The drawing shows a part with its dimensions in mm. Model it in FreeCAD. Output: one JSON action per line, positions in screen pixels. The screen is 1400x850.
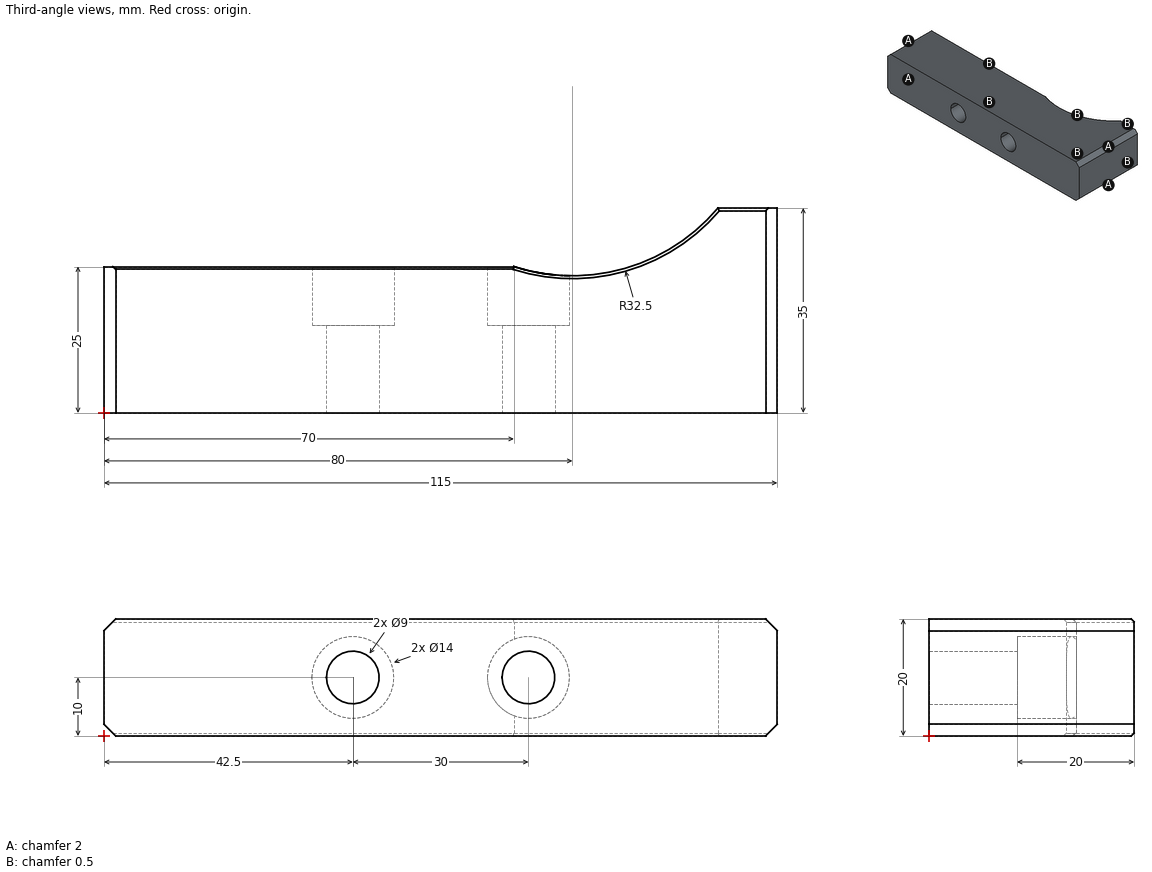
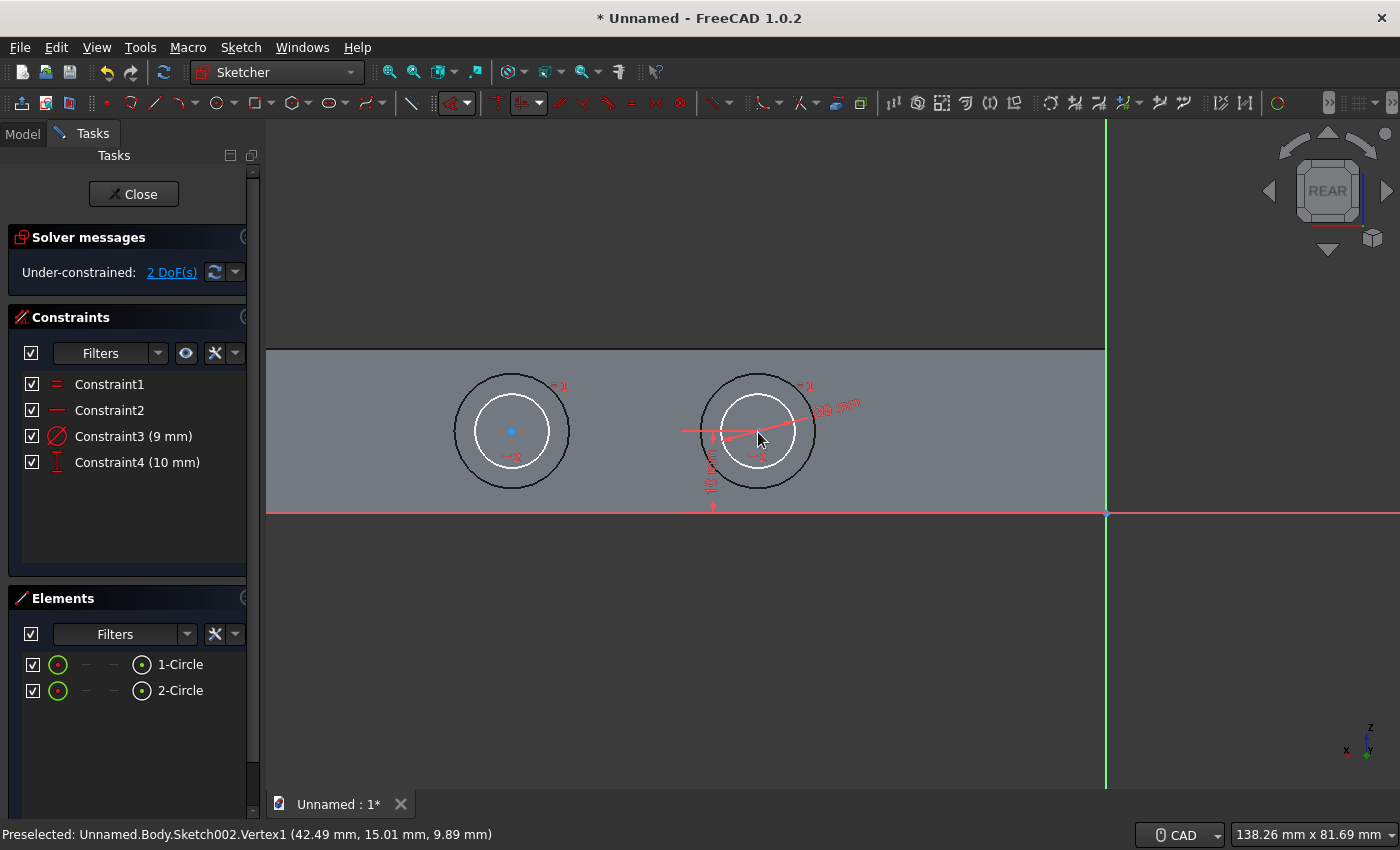
{"action": "left_click", "coordinate": [758, 431]}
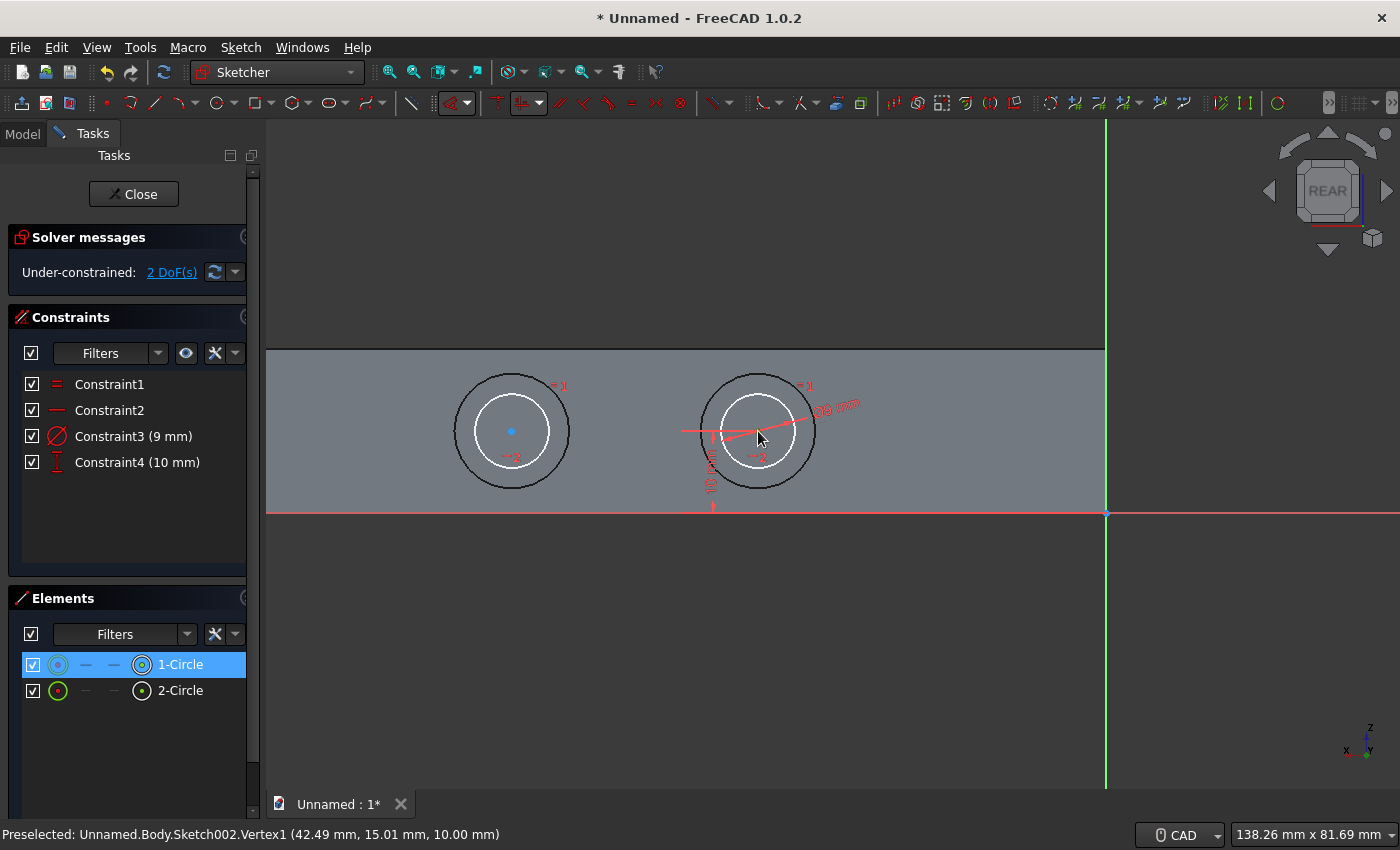
{"action": "left_click", "coordinate": [512, 431]}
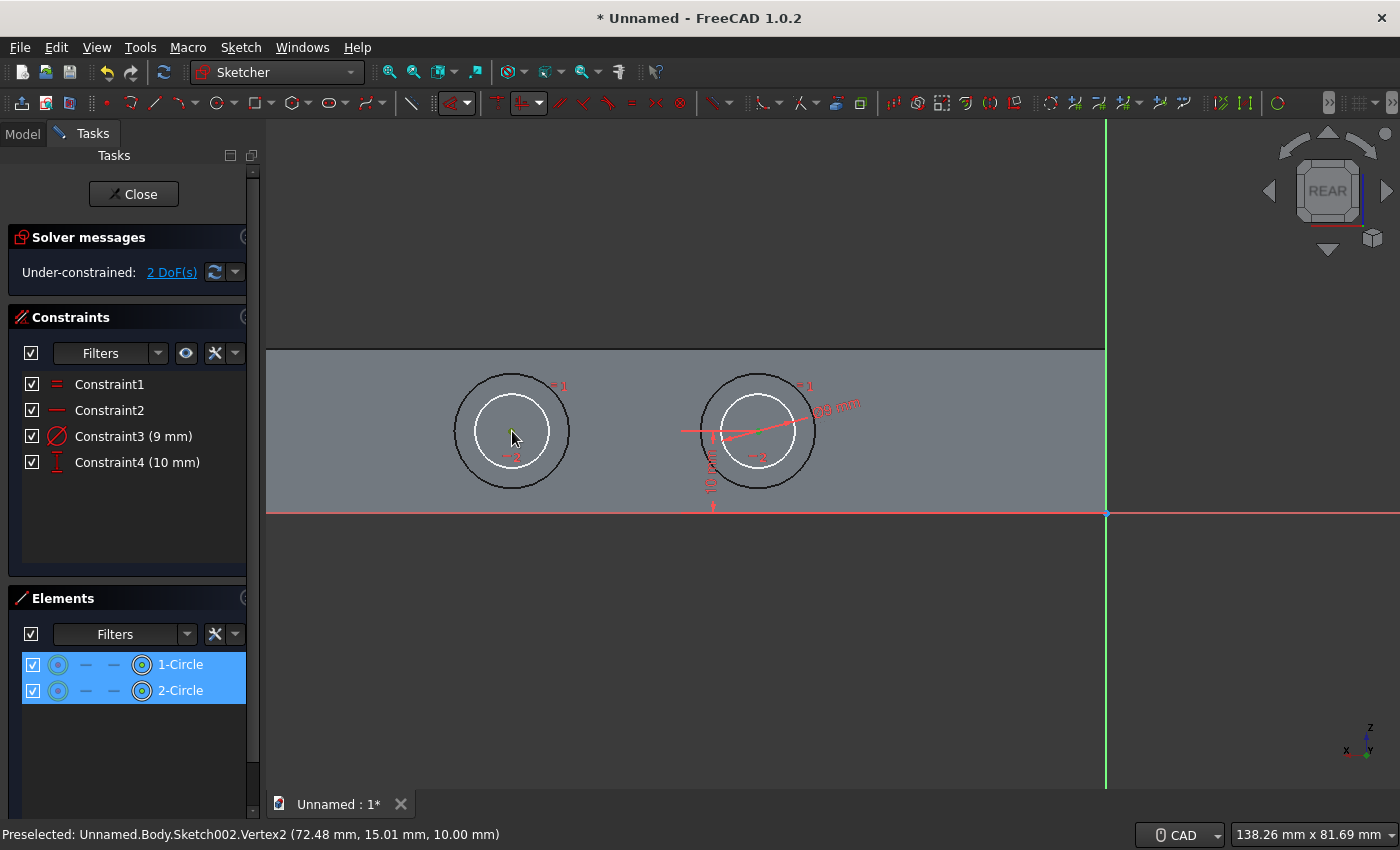
{"action": "left_click", "coordinate": [470, 104]}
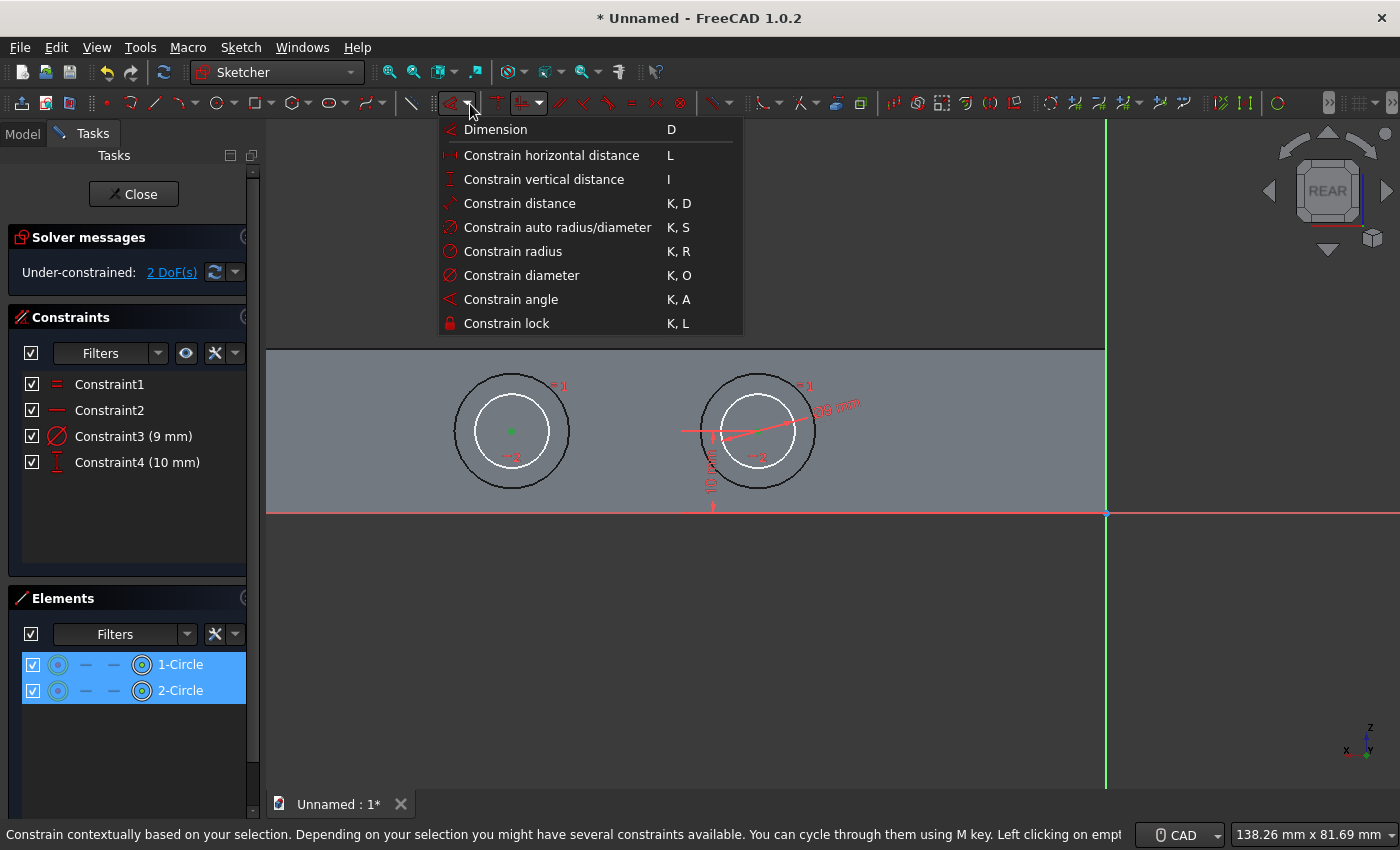
{"action": "left_click", "coordinate": [591, 155]}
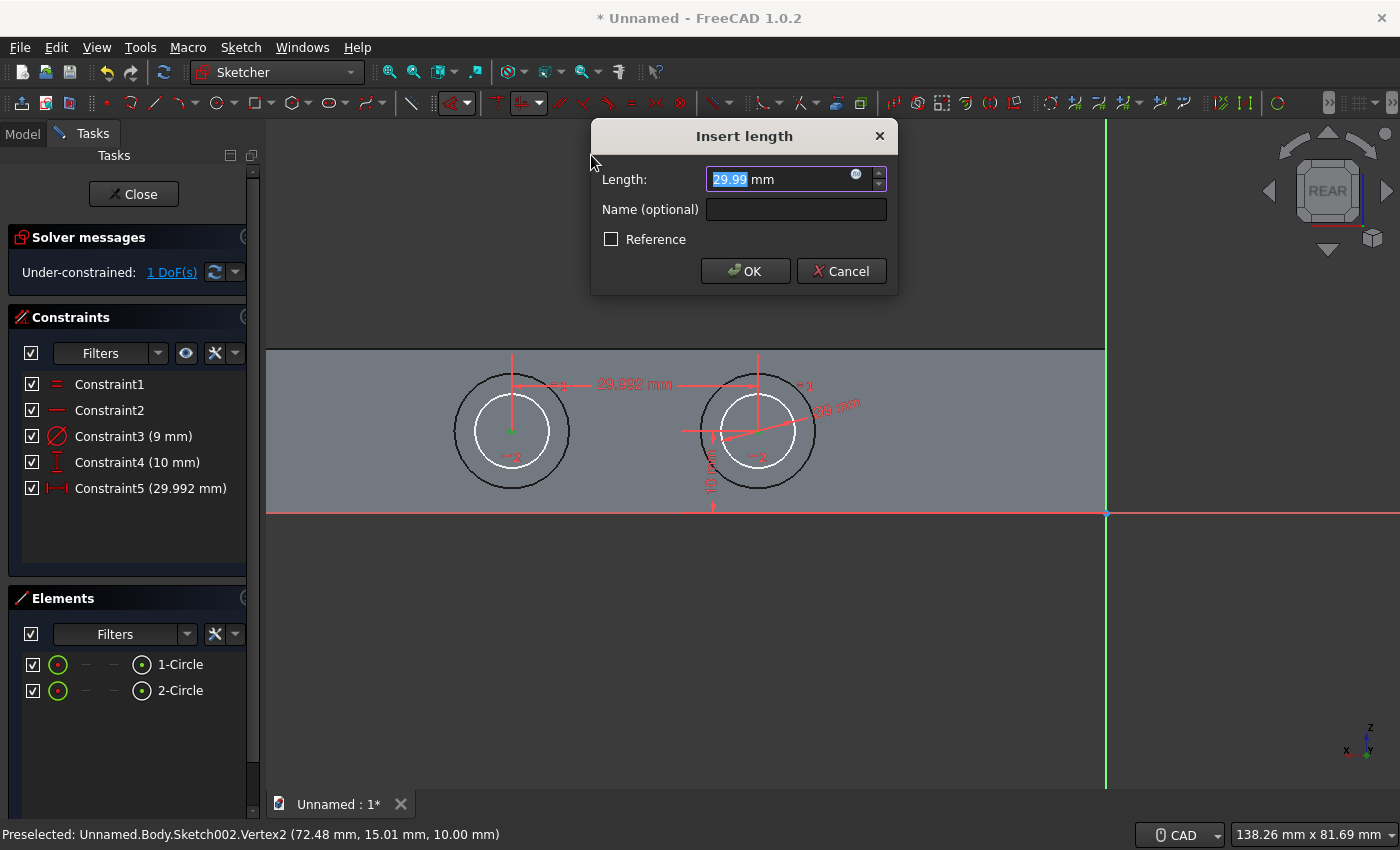
{"action": "type", "text": "30"}
{"action": "key", "text": "Return"}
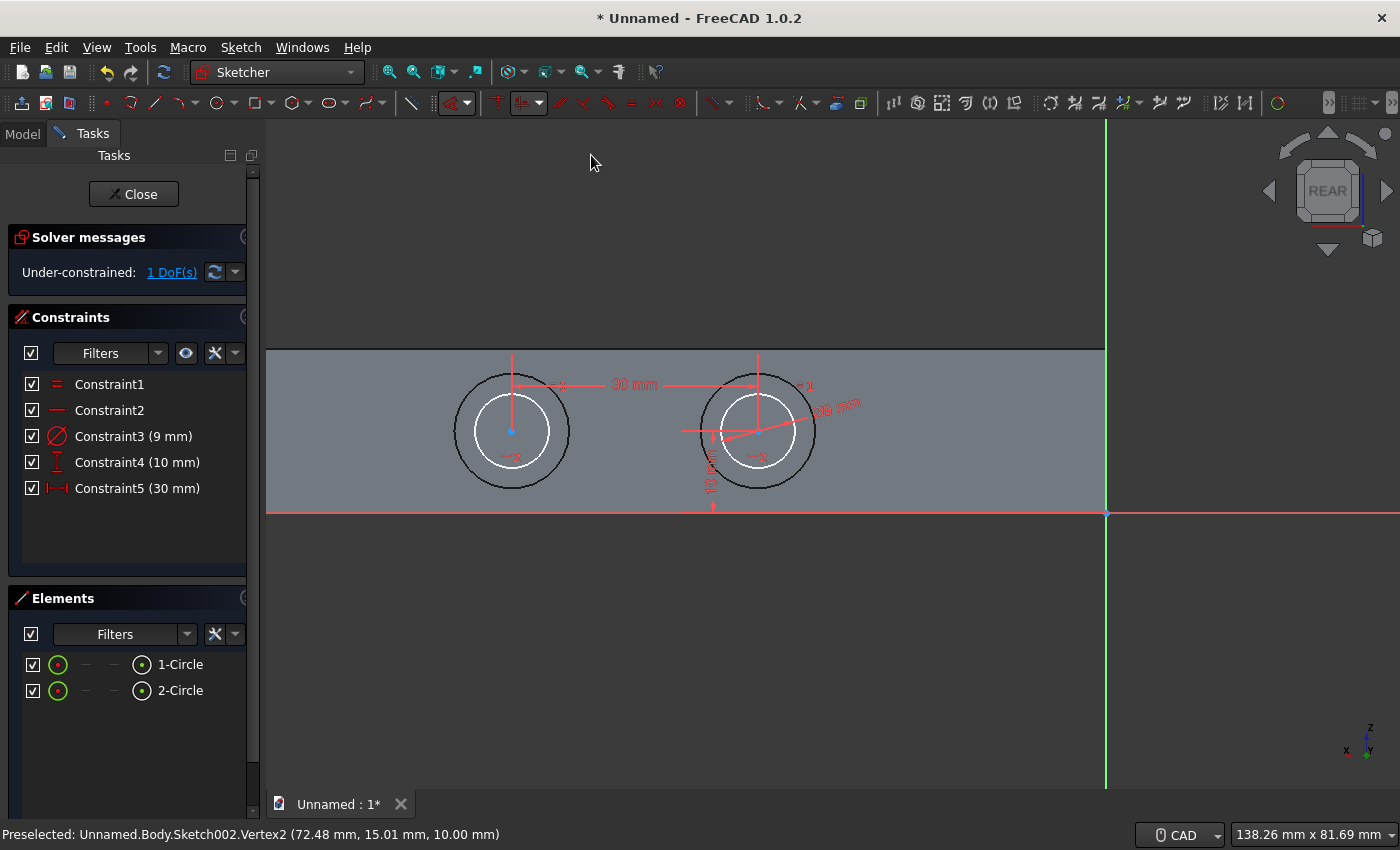
{"action": "left_click", "coordinate": [758, 431]}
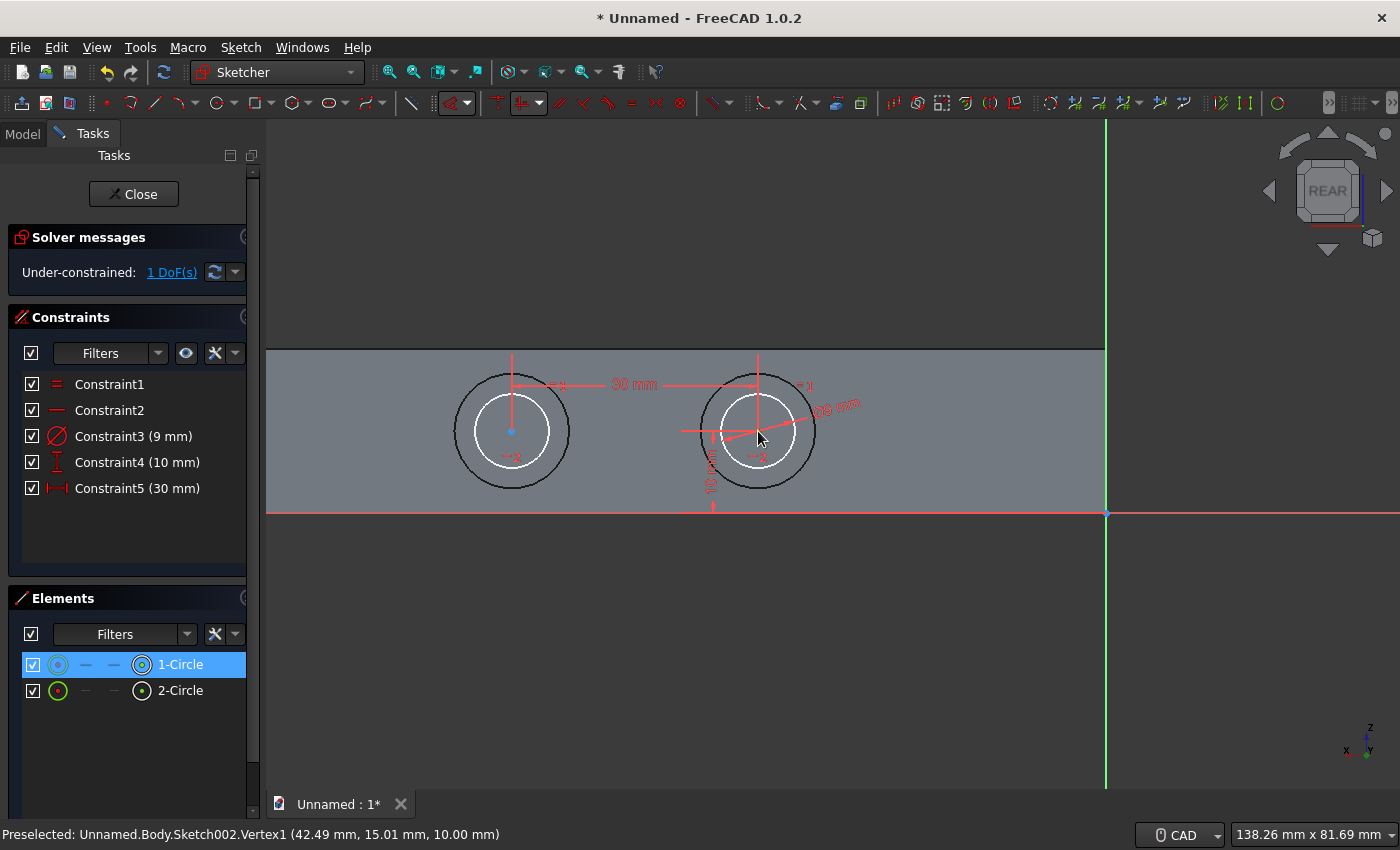
{"action": "key", "text": "l"}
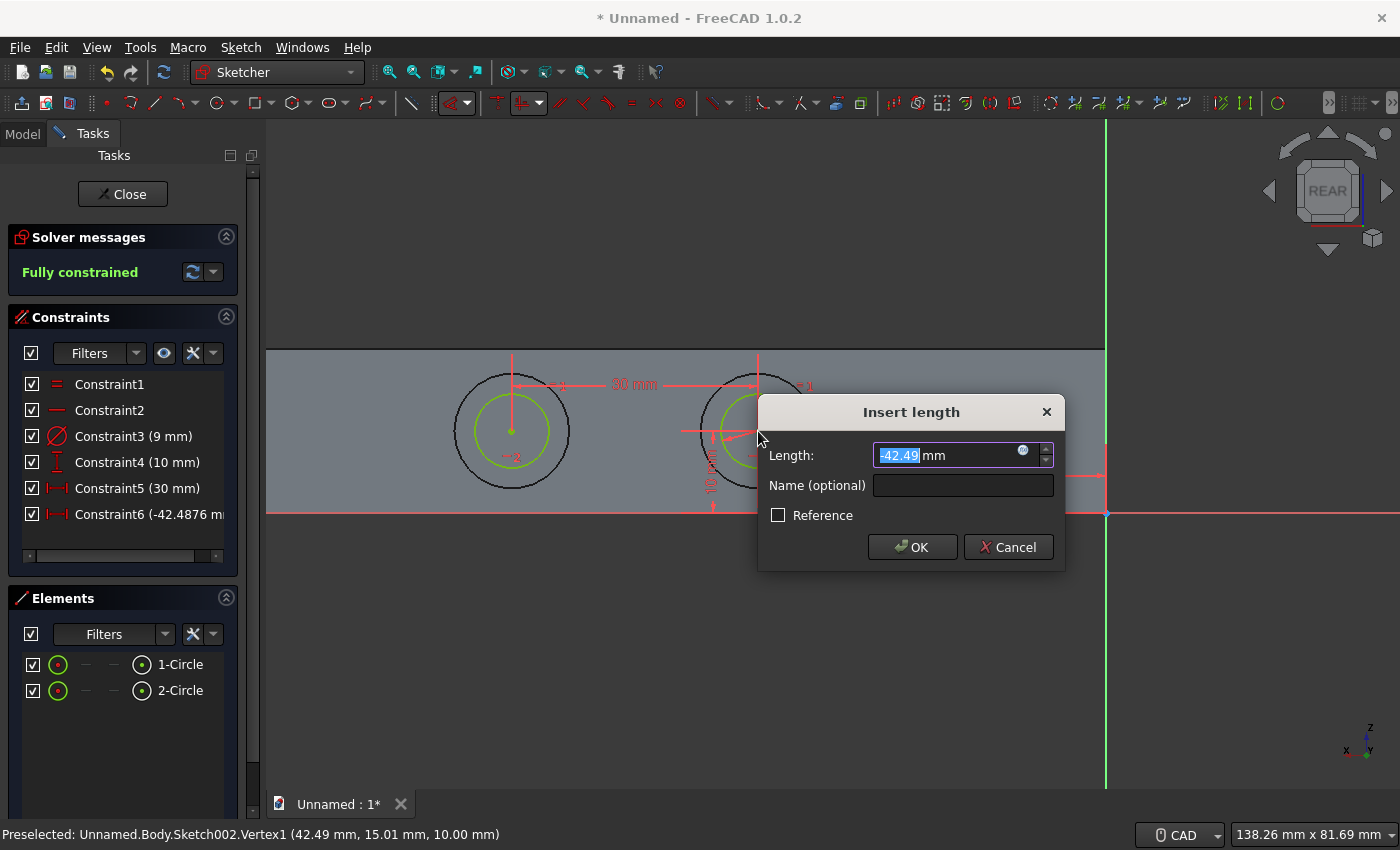
{"action": "type", "text": "-42.5"}
{"action": "key", "text": "Return"}